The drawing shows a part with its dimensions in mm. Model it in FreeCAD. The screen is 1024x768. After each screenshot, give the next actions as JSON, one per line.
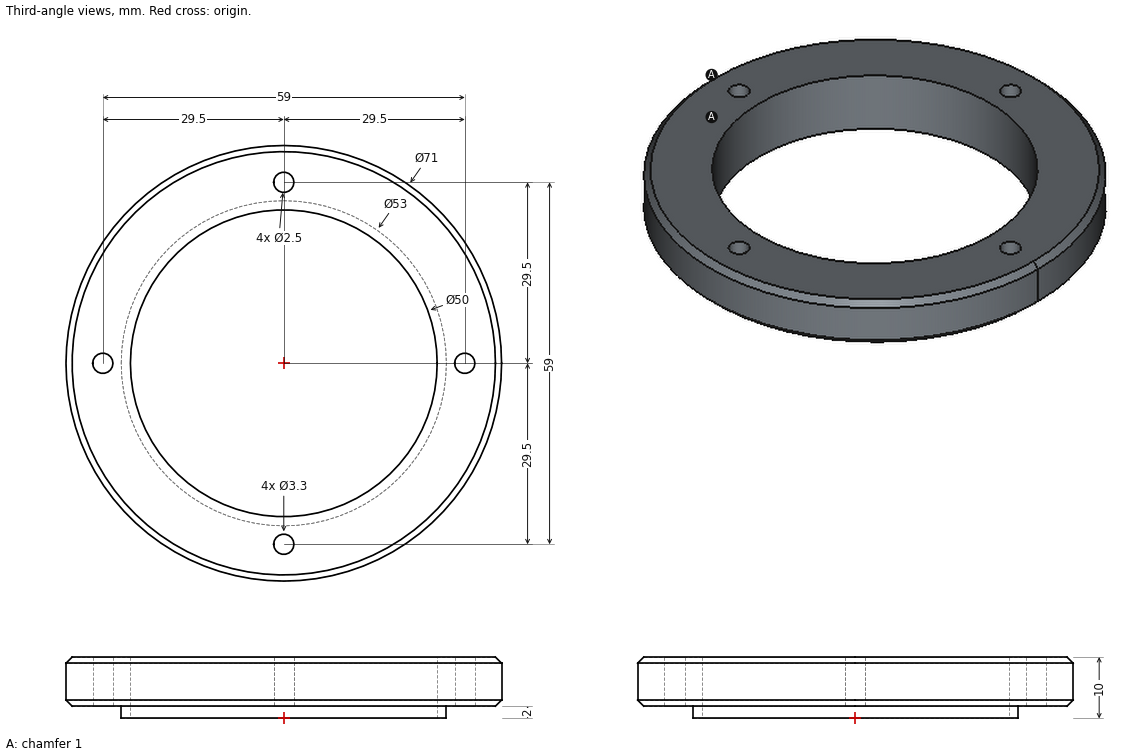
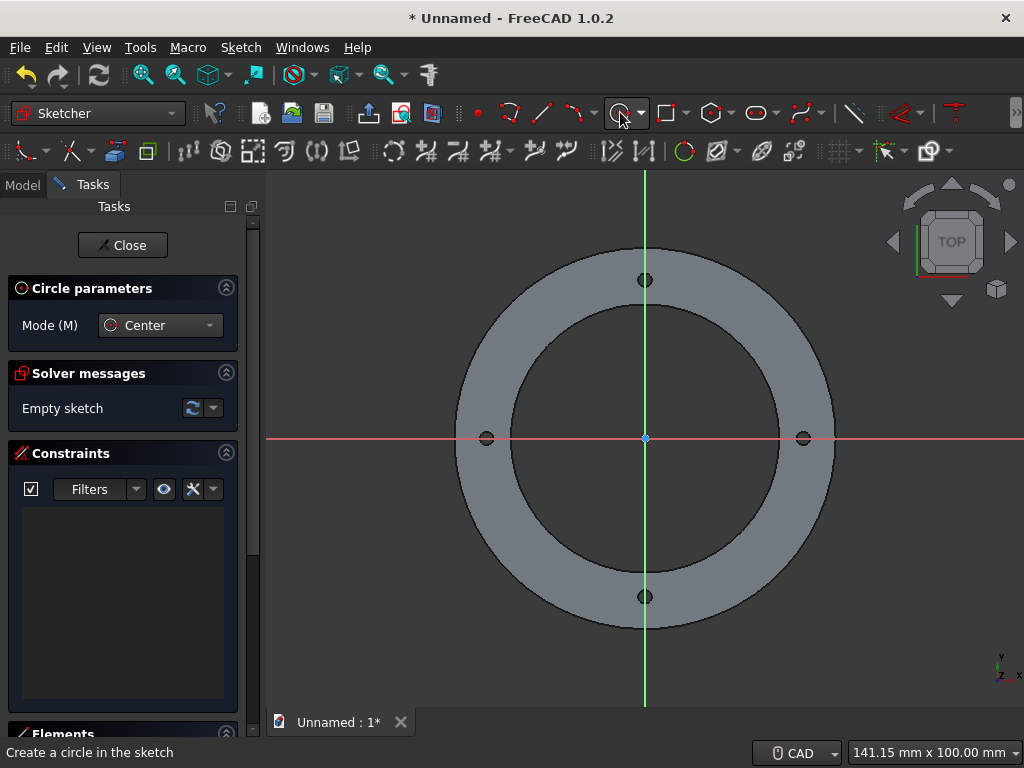
{"action": "scroll", "coordinate": [645, 597], "scroll_direction": "up", "scroll_amount": 5}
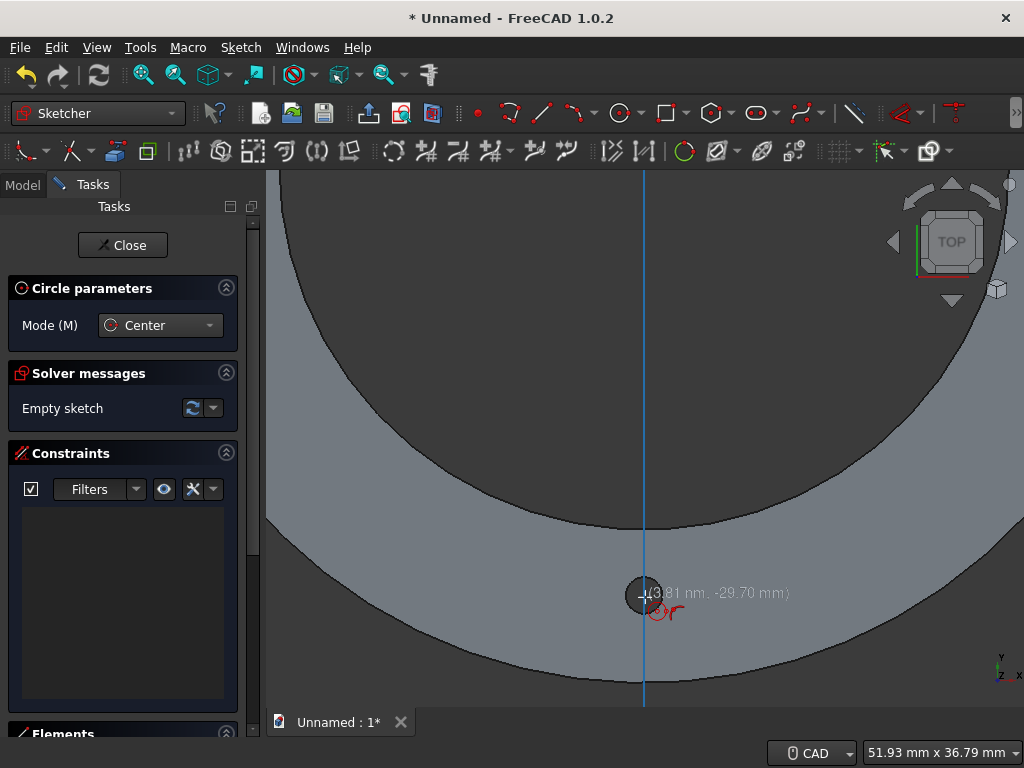
{"action": "left_click", "coordinate": [644, 595]}
{"action": "mouse_move", "coordinate": [661, 578]}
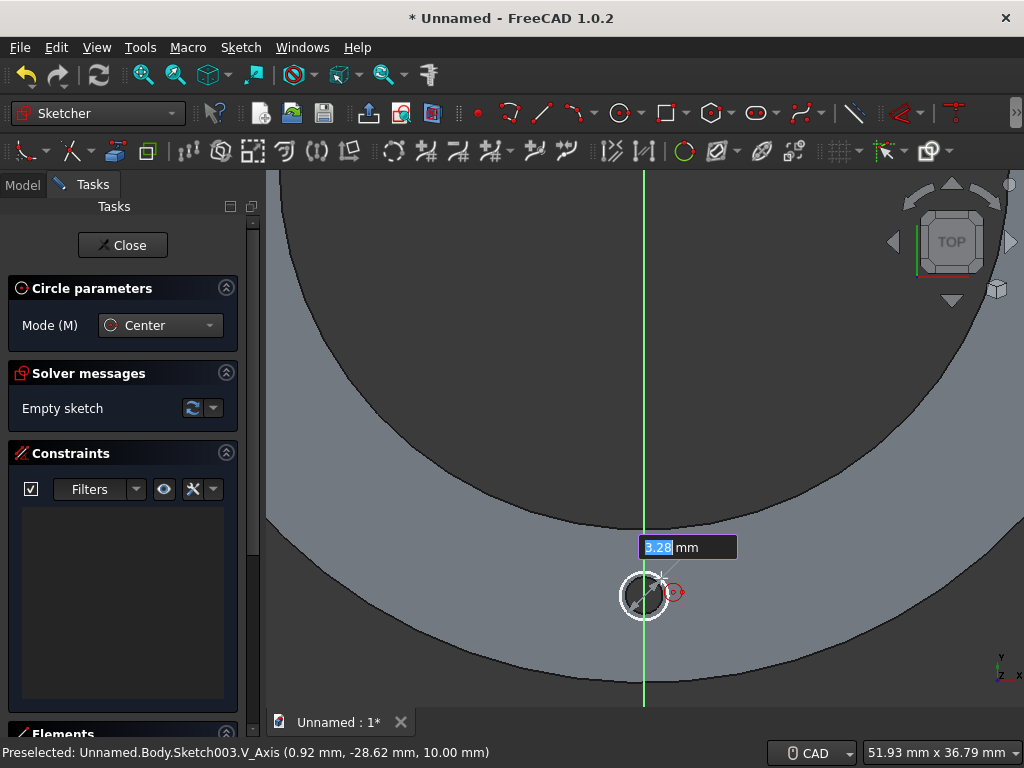
{"action": "type", "text": "3.3"}
{"action": "key", "text": "Return"}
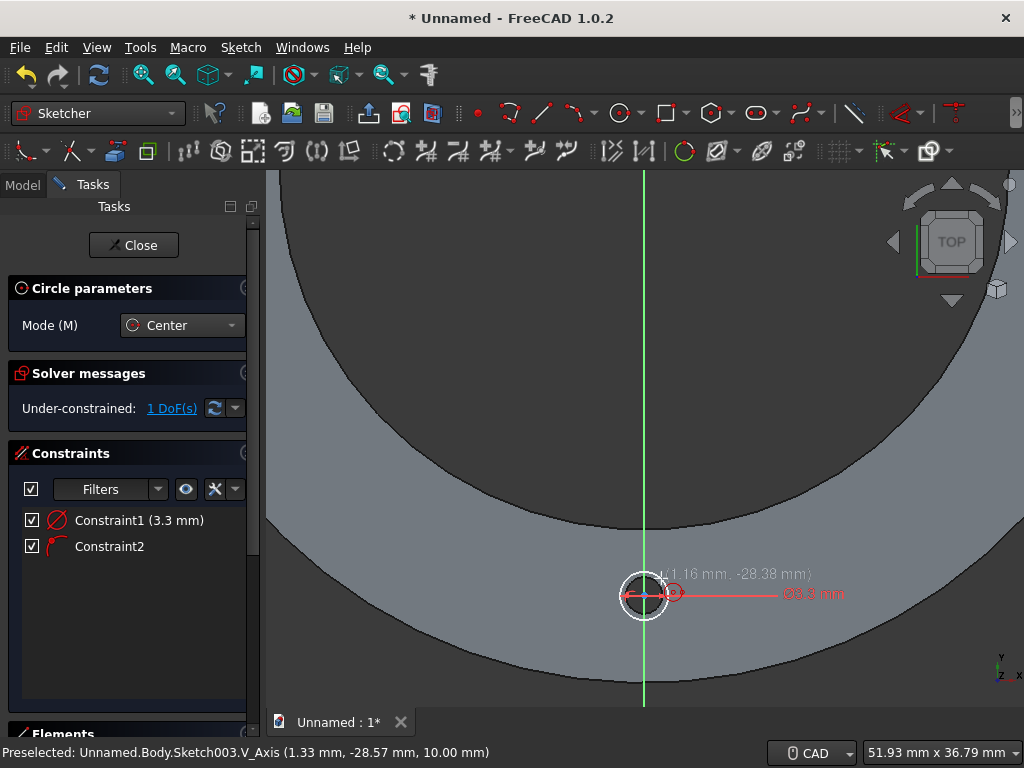
{"action": "scroll", "coordinate": [537, 598], "scroll_direction": "down", "scroll_amount": 5}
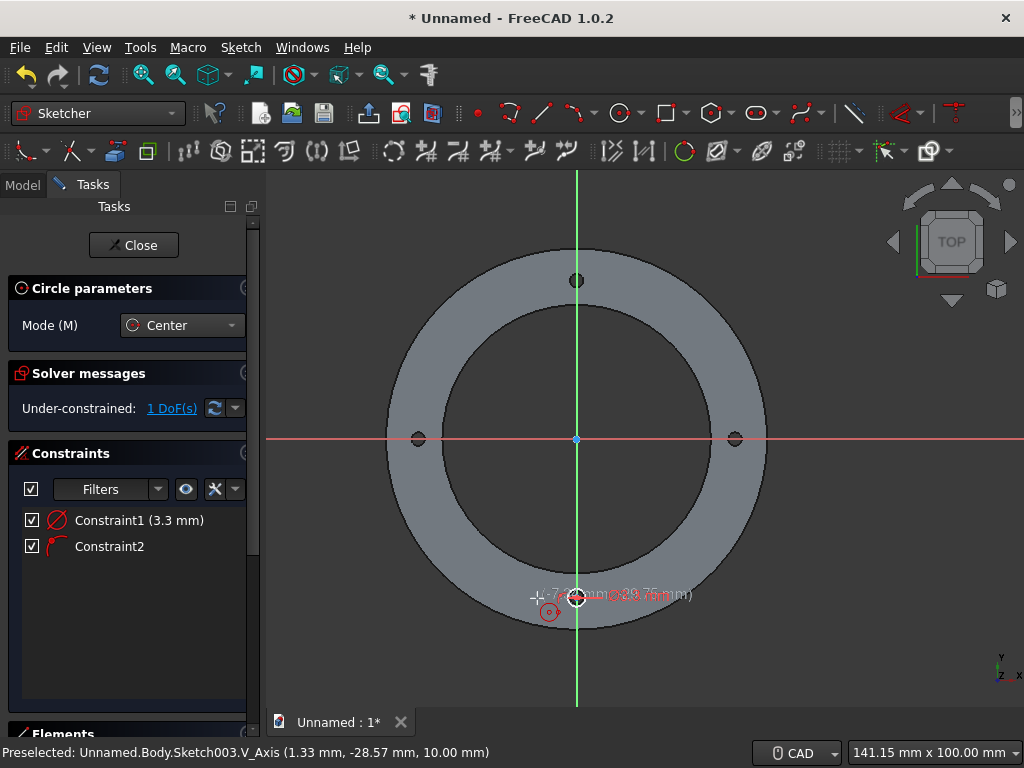
{"action": "scroll", "coordinate": [418, 439], "scroll_direction": "up", "scroll_amount": 5}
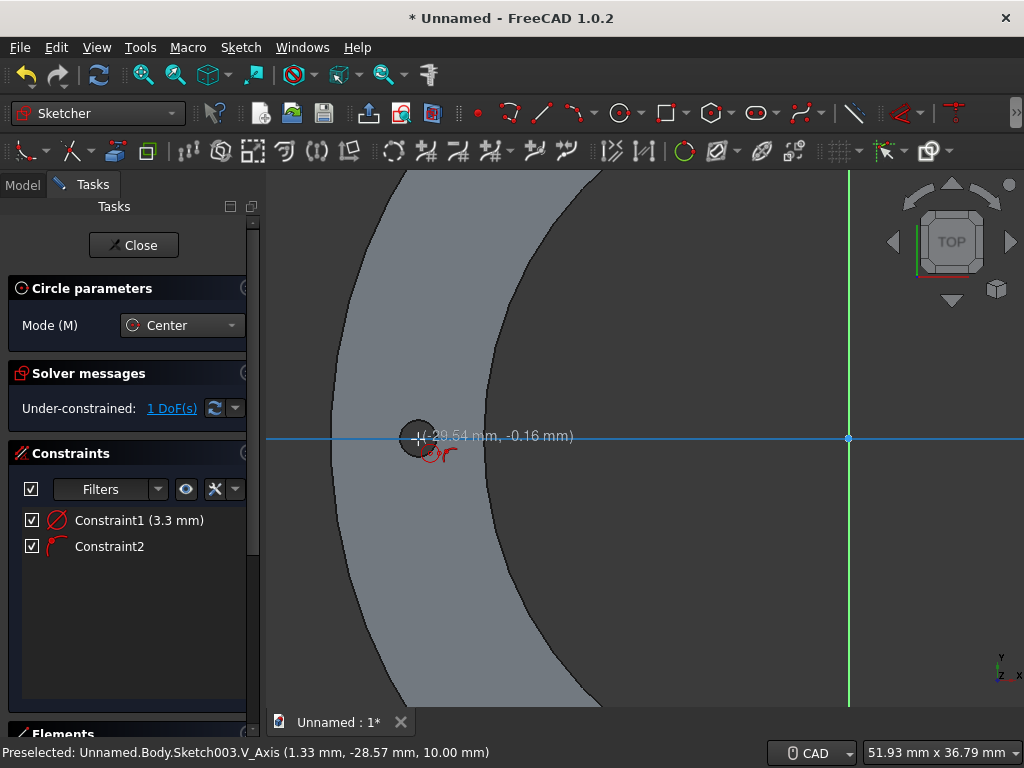
{"action": "left_click", "coordinate": [418, 438]}
{"action": "mouse_move", "coordinate": [435, 421]}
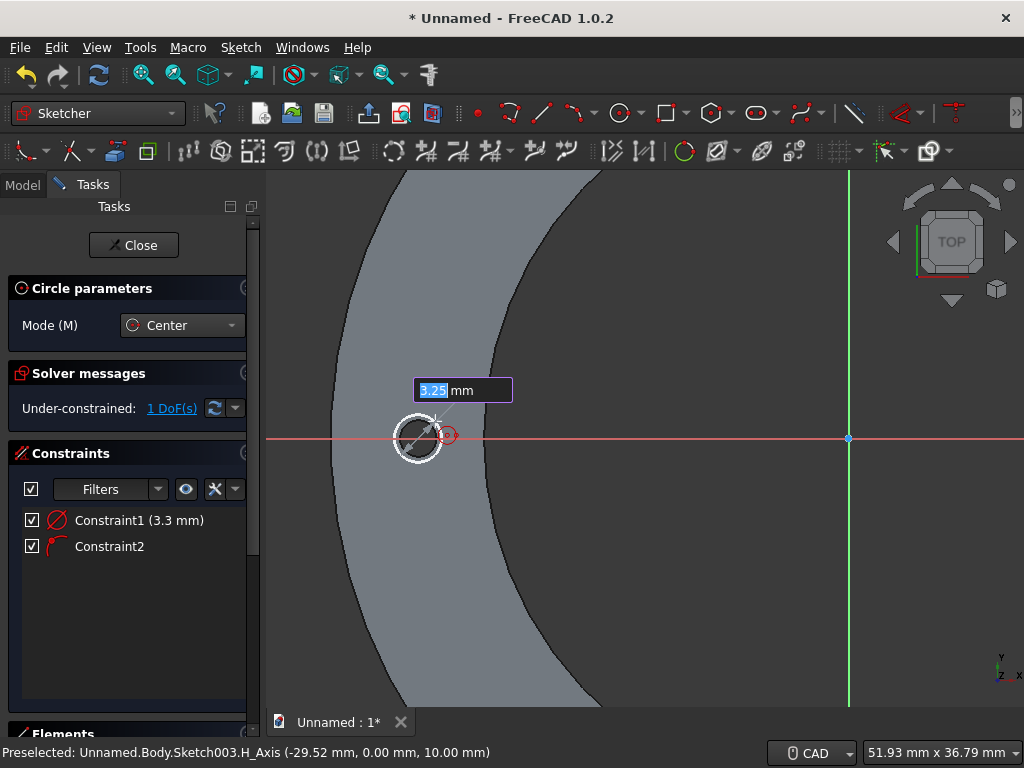
{"action": "type", "text": "3.3"}
{"action": "key", "text": "Return"}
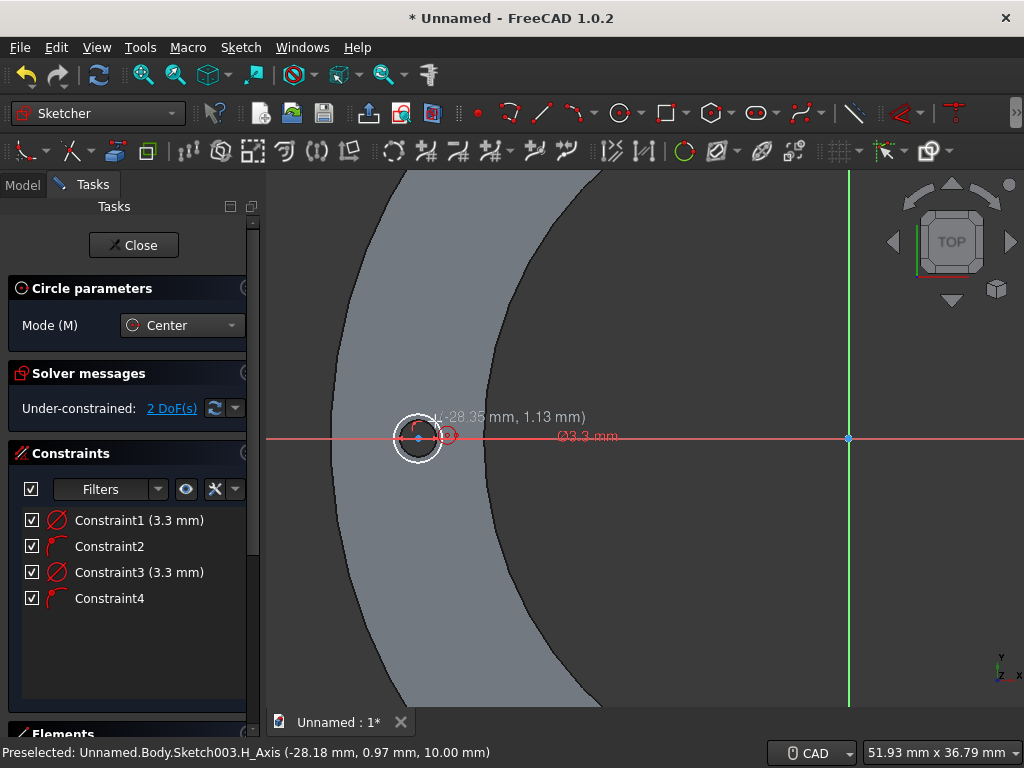
{"action": "scroll", "coordinate": [418, 439], "scroll_direction": "down", "scroll_amount": 5}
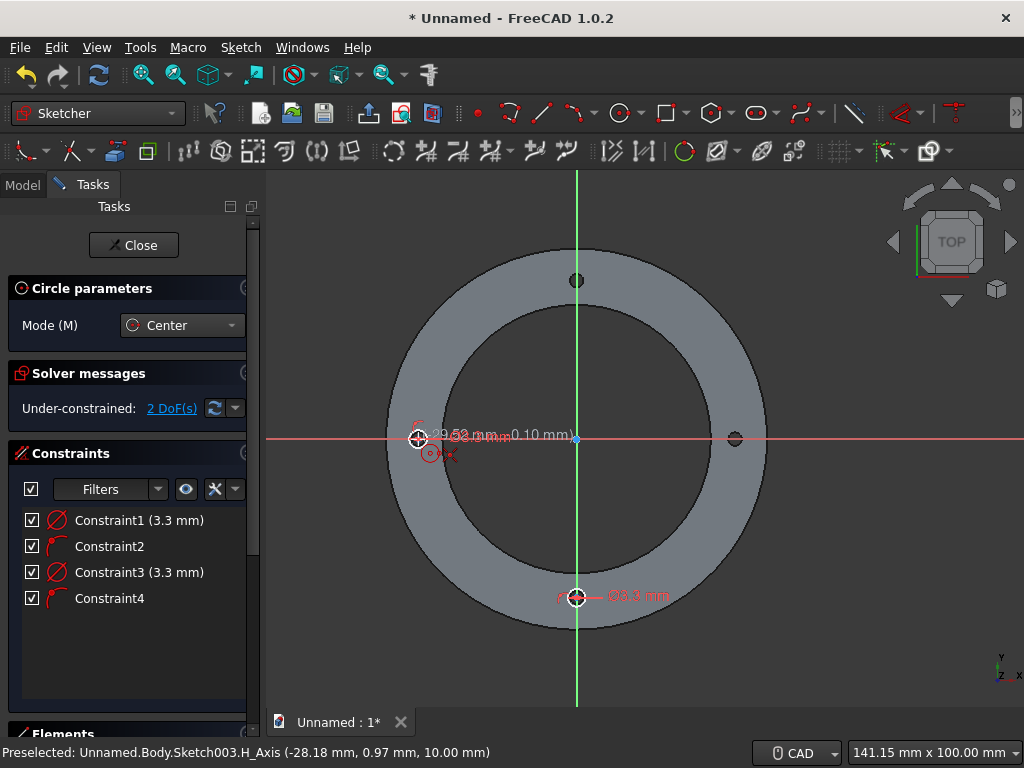
{"action": "scroll", "coordinate": [577, 281], "scroll_direction": "up", "scroll_amount": 5}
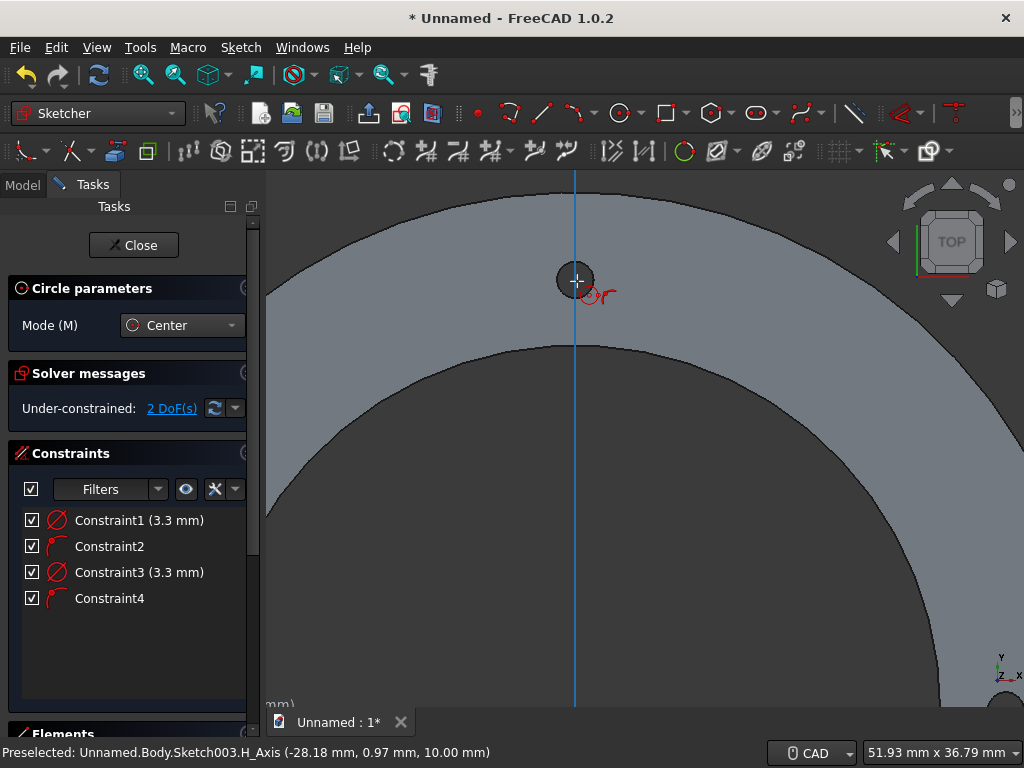
{"action": "left_click", "coordinate": [575, 280]}
{"action": "mouse_move", "coordinate": [592, 263]}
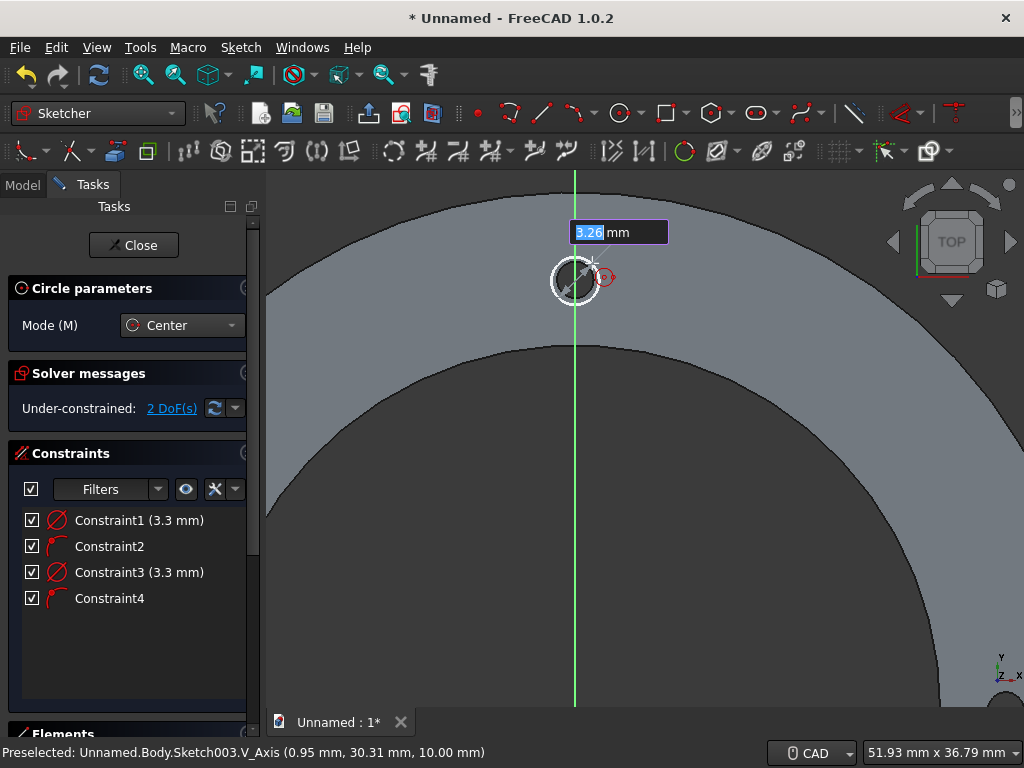
{"action": "type", "text": "3.3"}
{"action": "key", "text": "Return"}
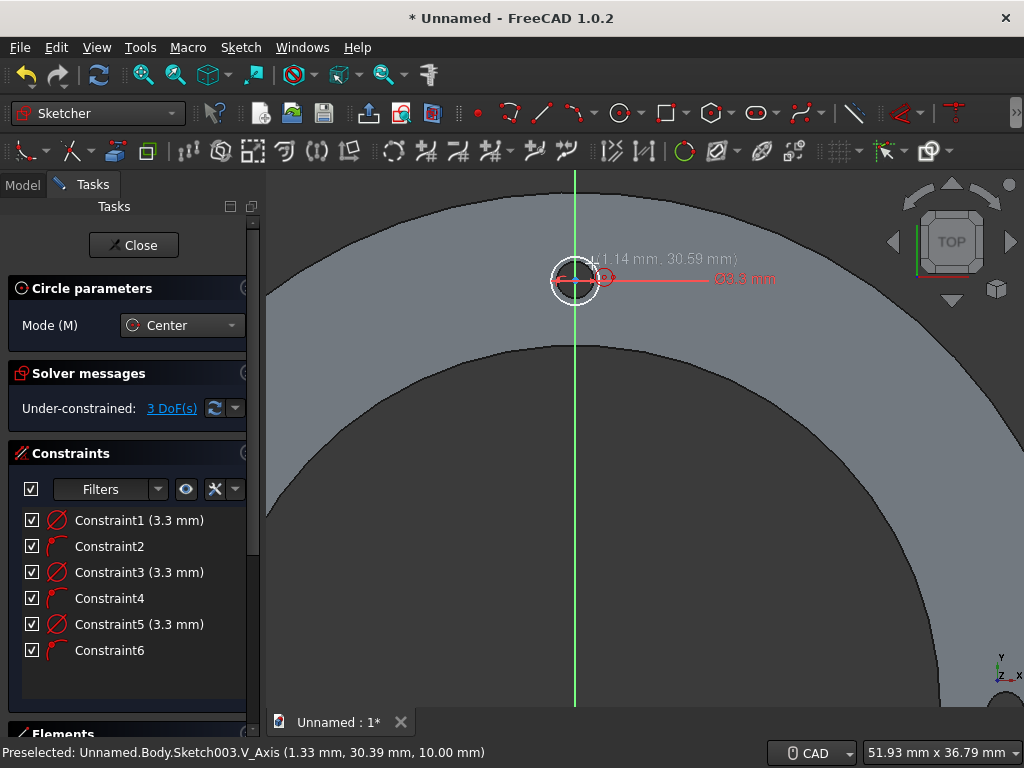
{"action": "scroll", "coordinate": [577, 280], "scroll_direction": "down", "scroll_amount": 5}